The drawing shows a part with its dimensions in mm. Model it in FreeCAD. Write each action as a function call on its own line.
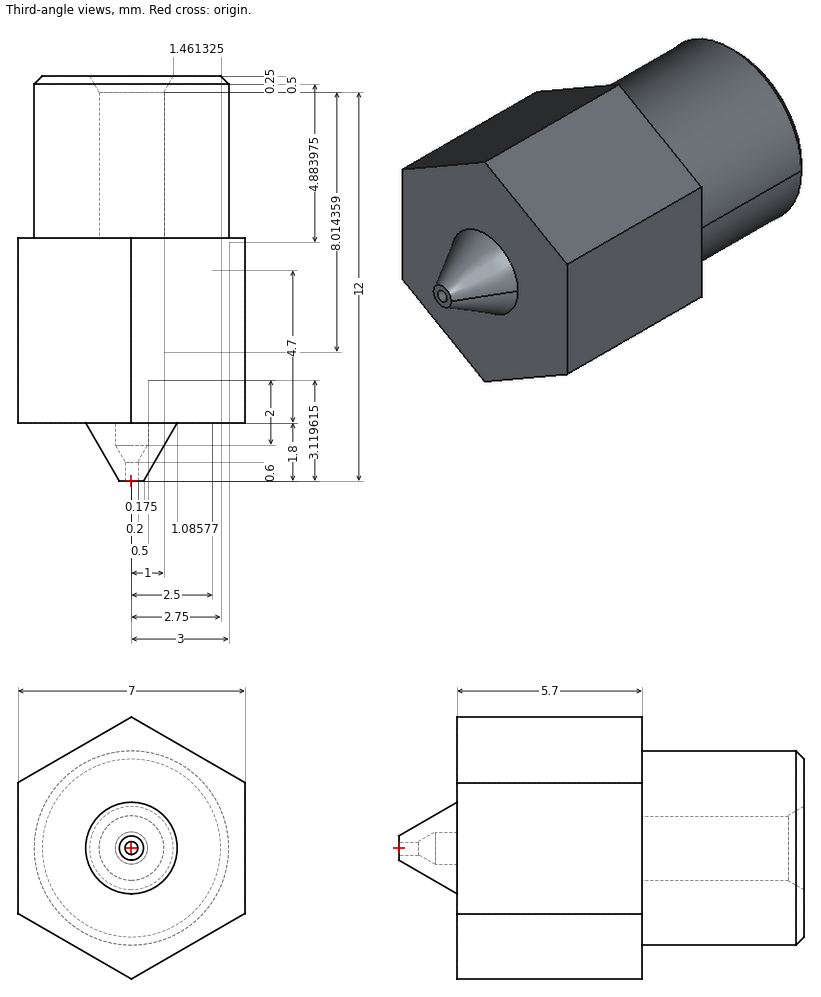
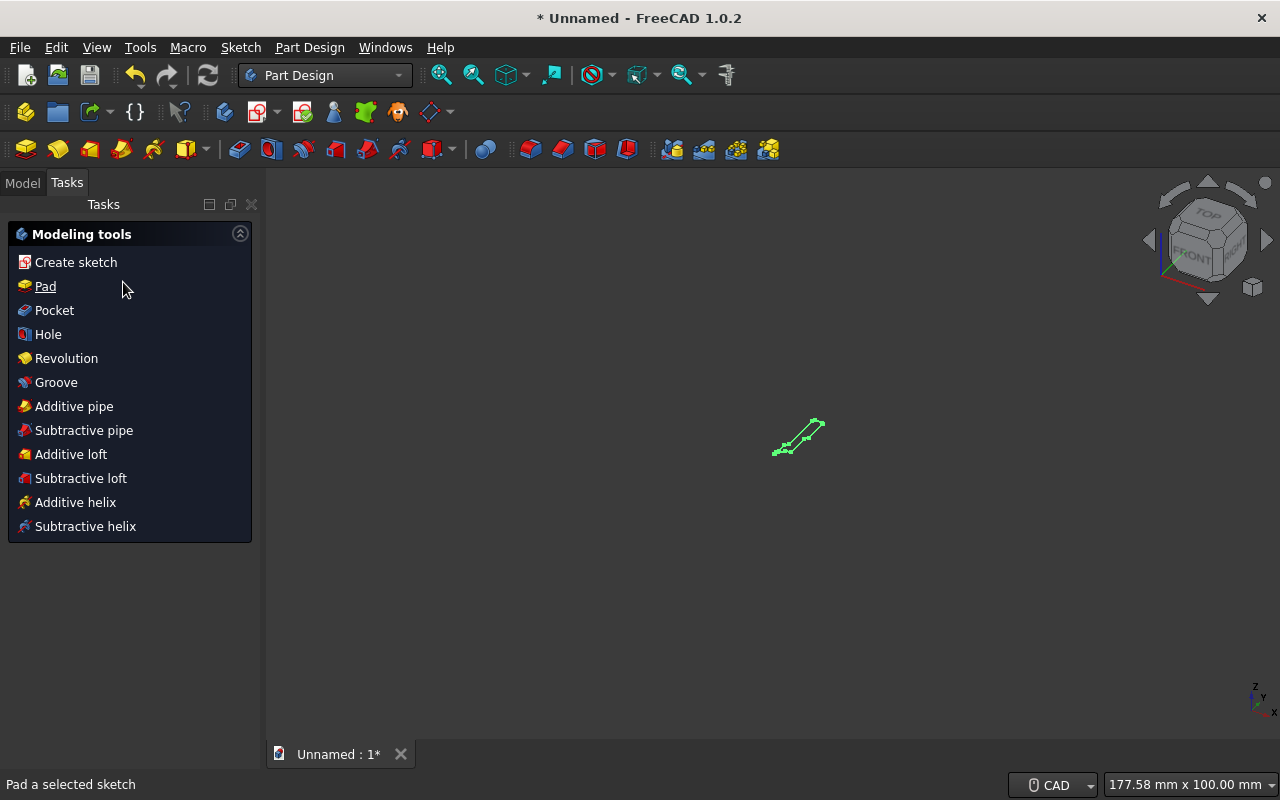
click(58, 150)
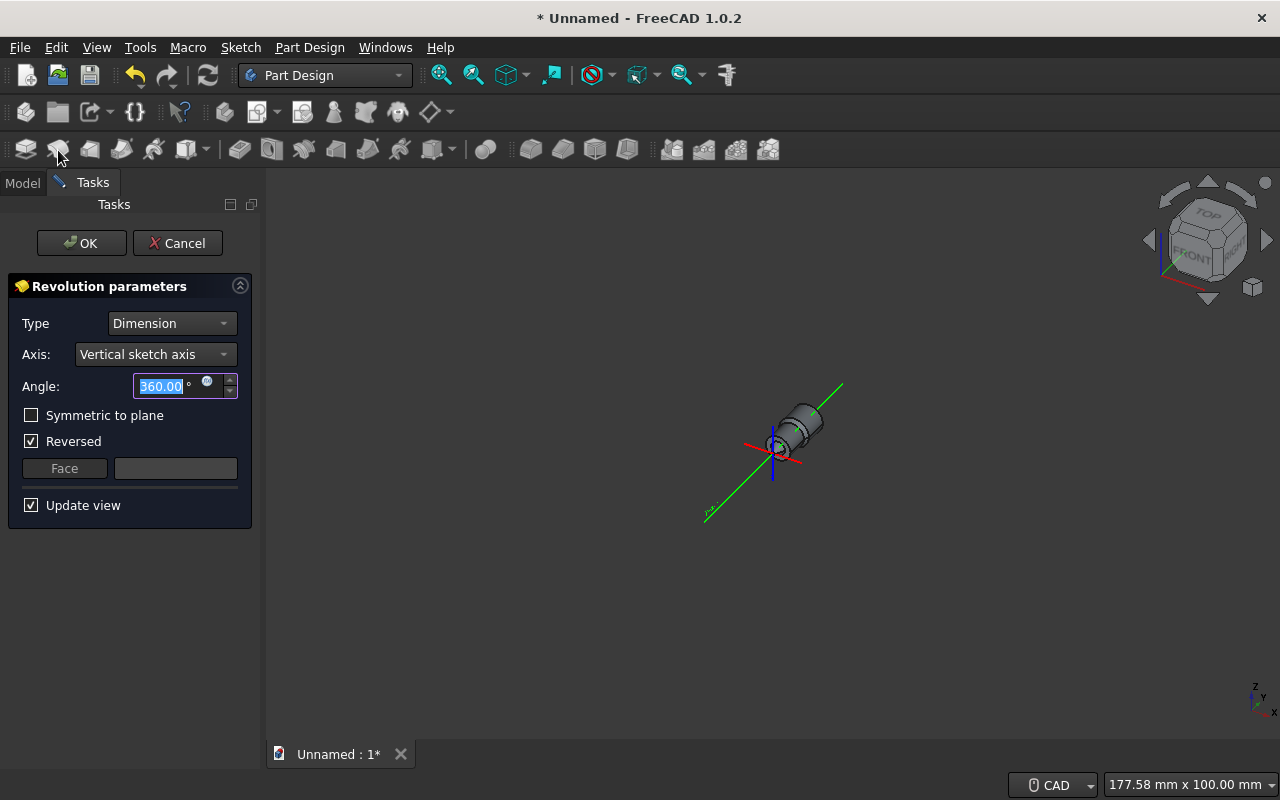
click(82, 243)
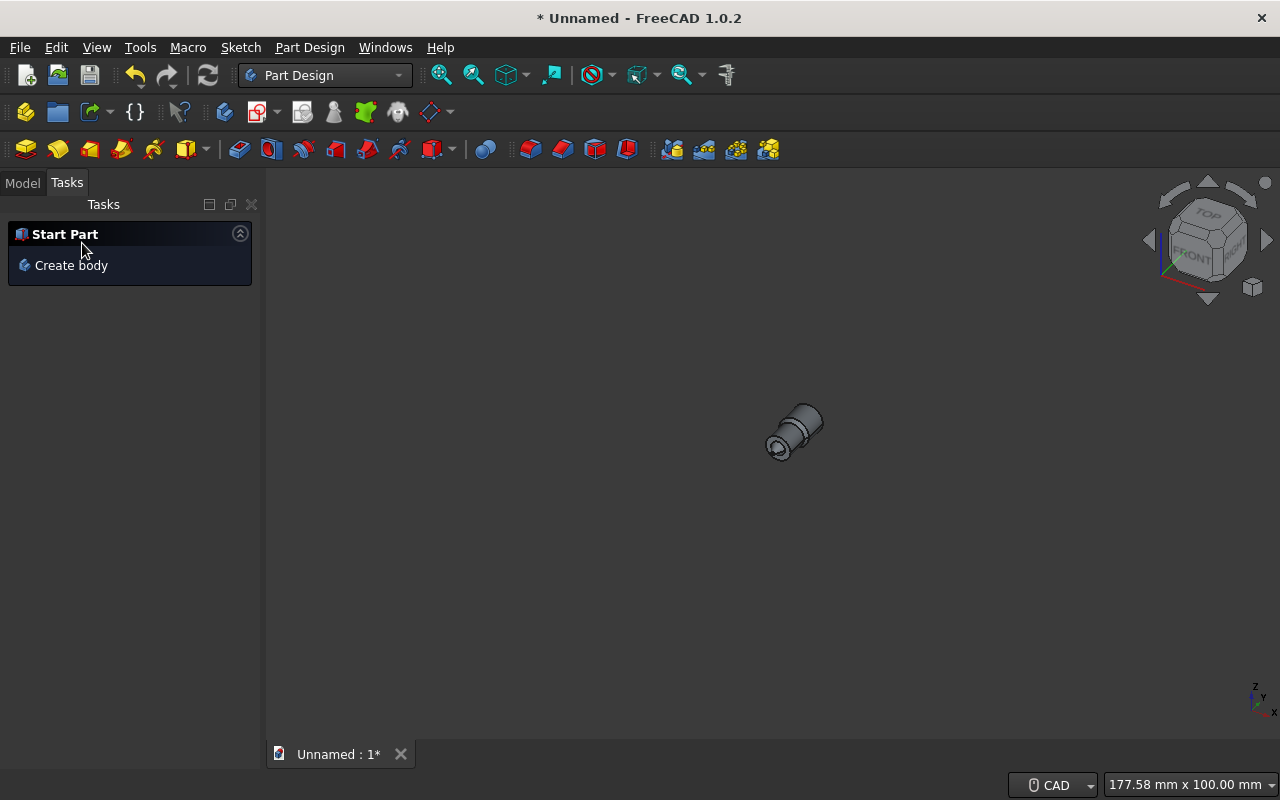
click(442, 76)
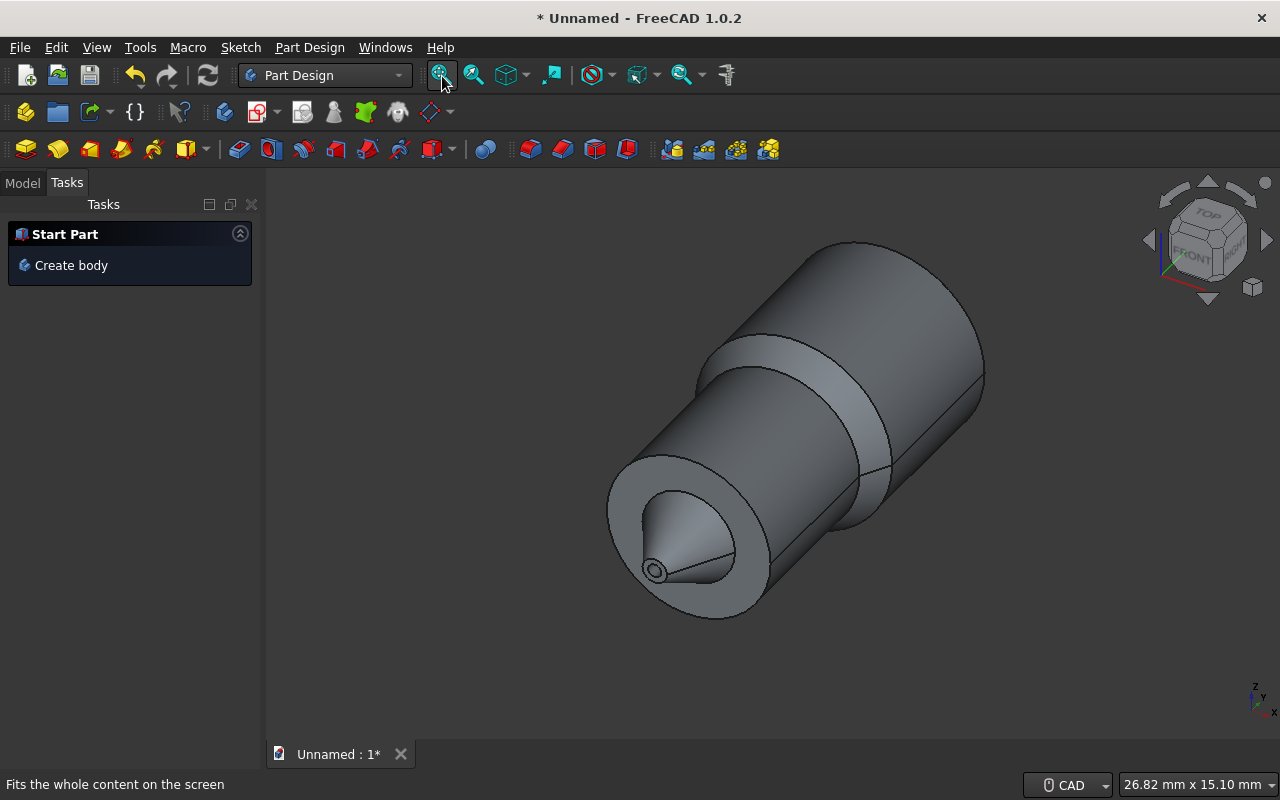
click(736, 507)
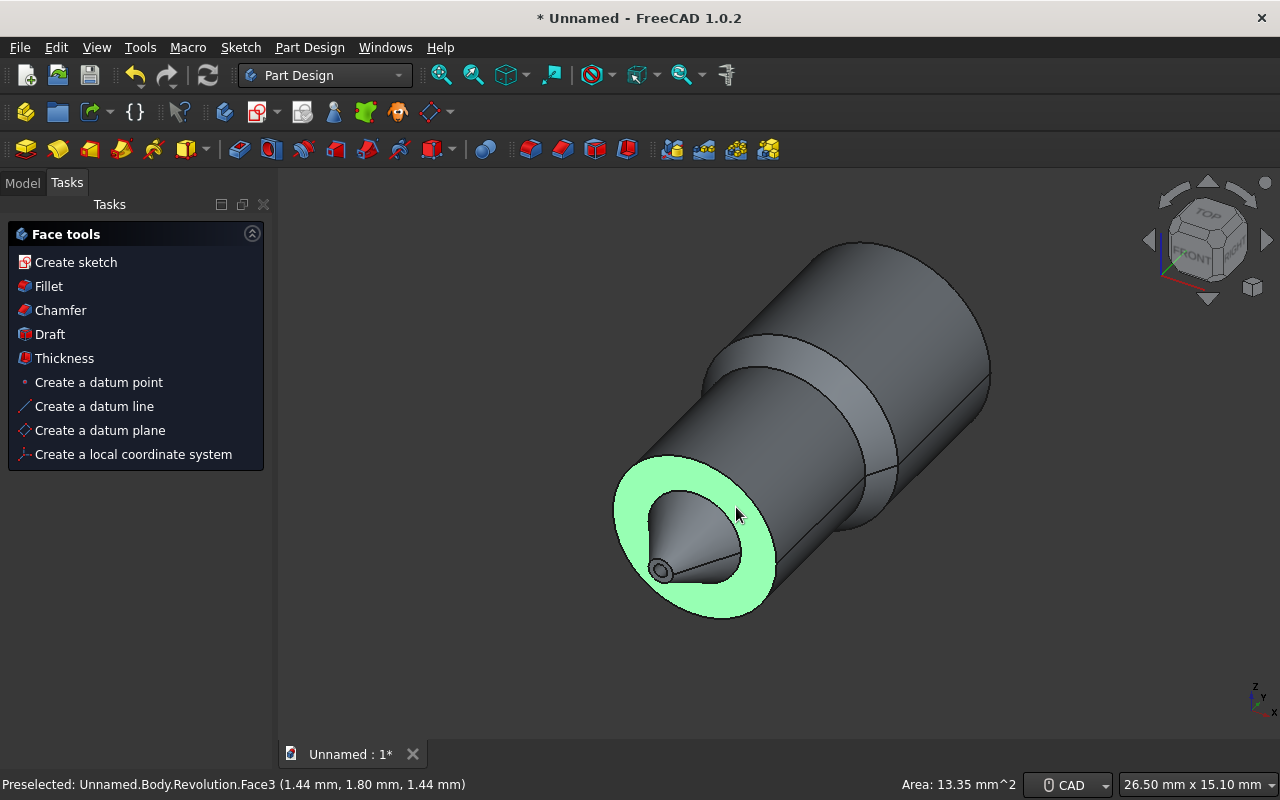
click(258, 112)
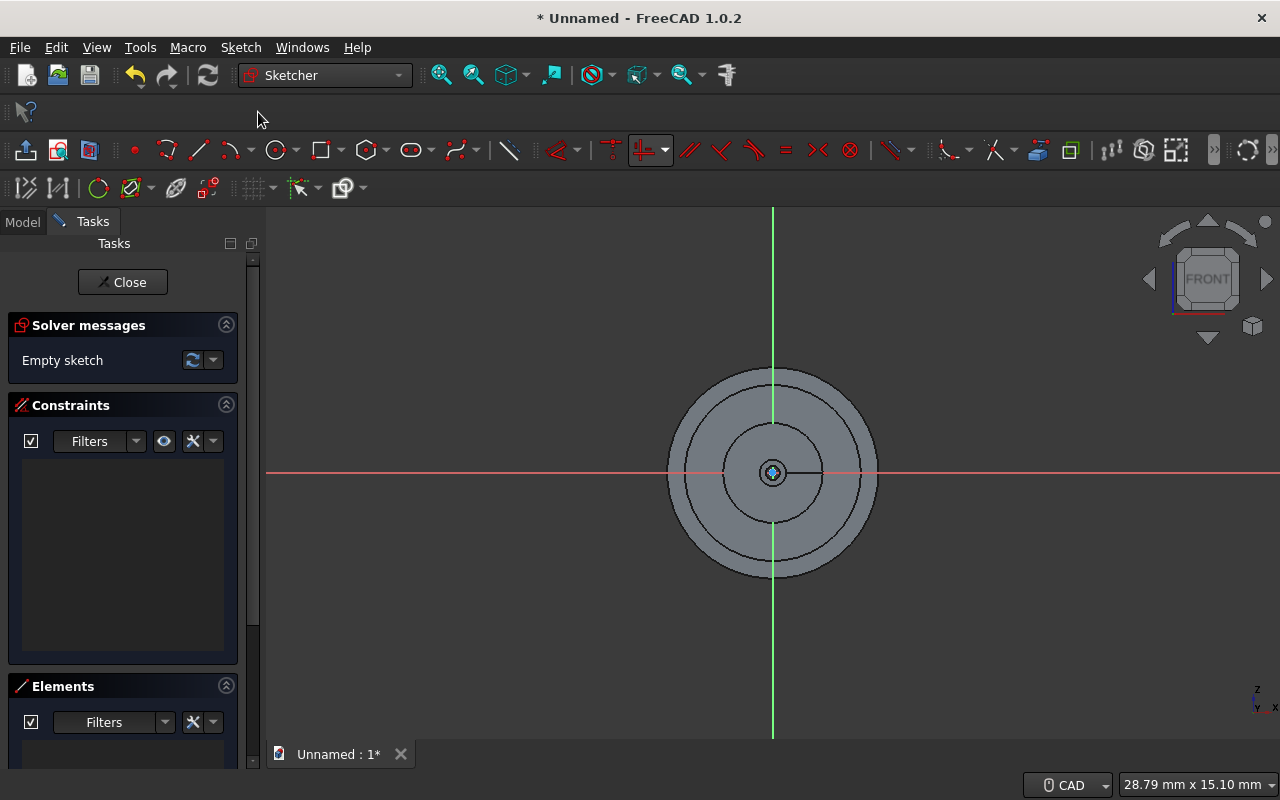
click(366, 150)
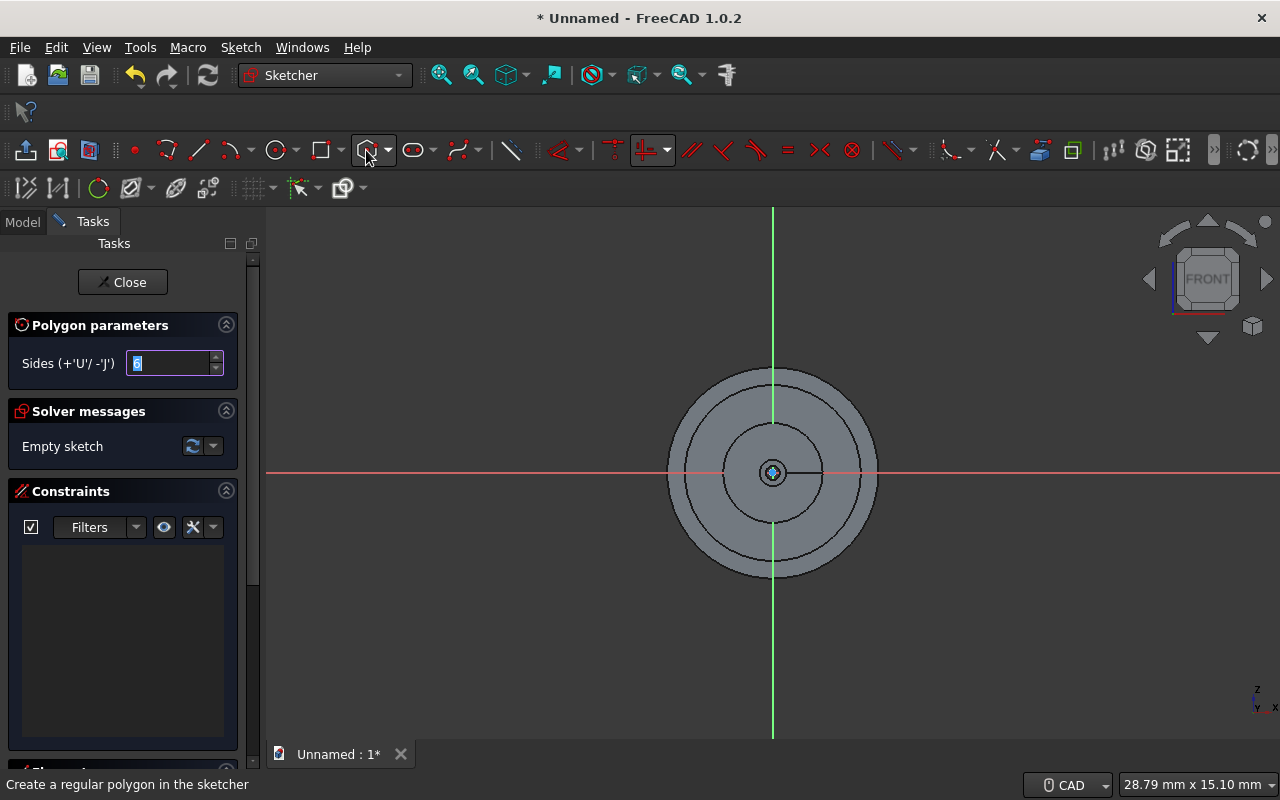
click(773, 473)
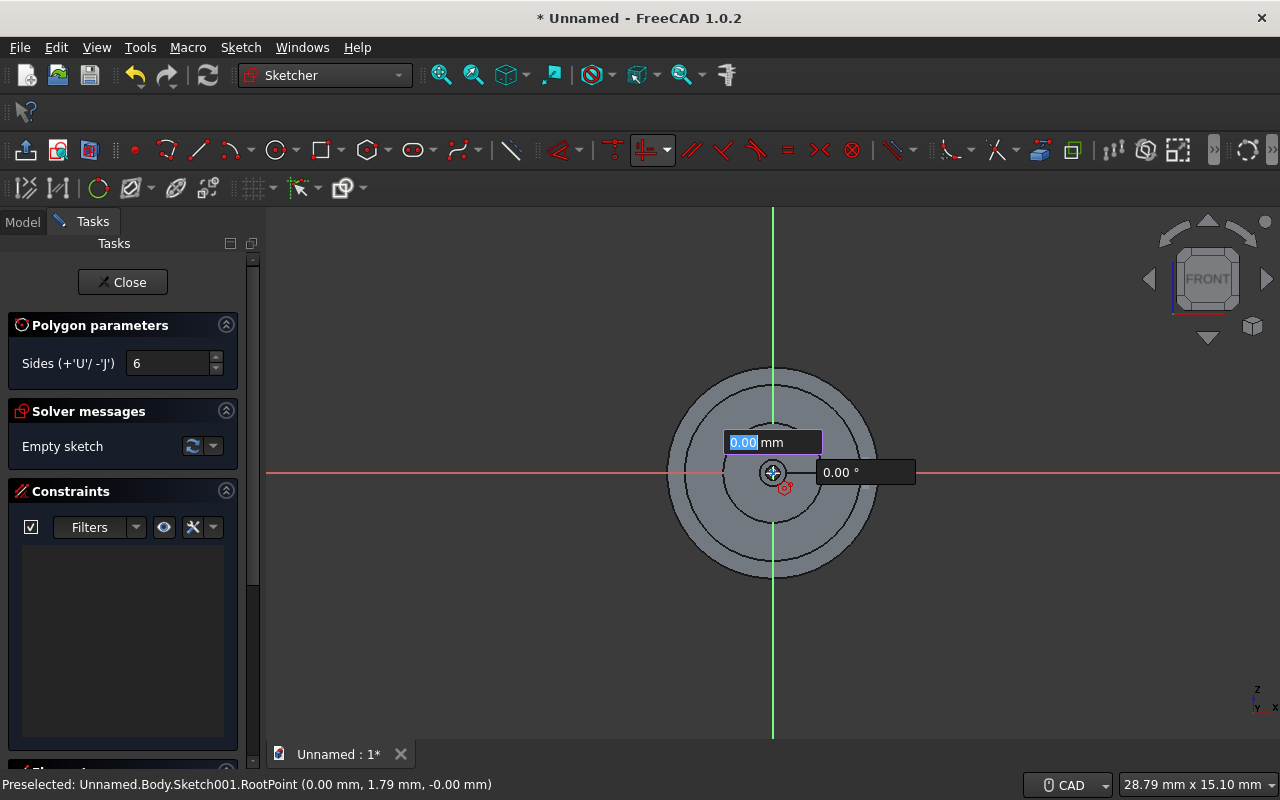
click(773, 331)
right_click(773, 331)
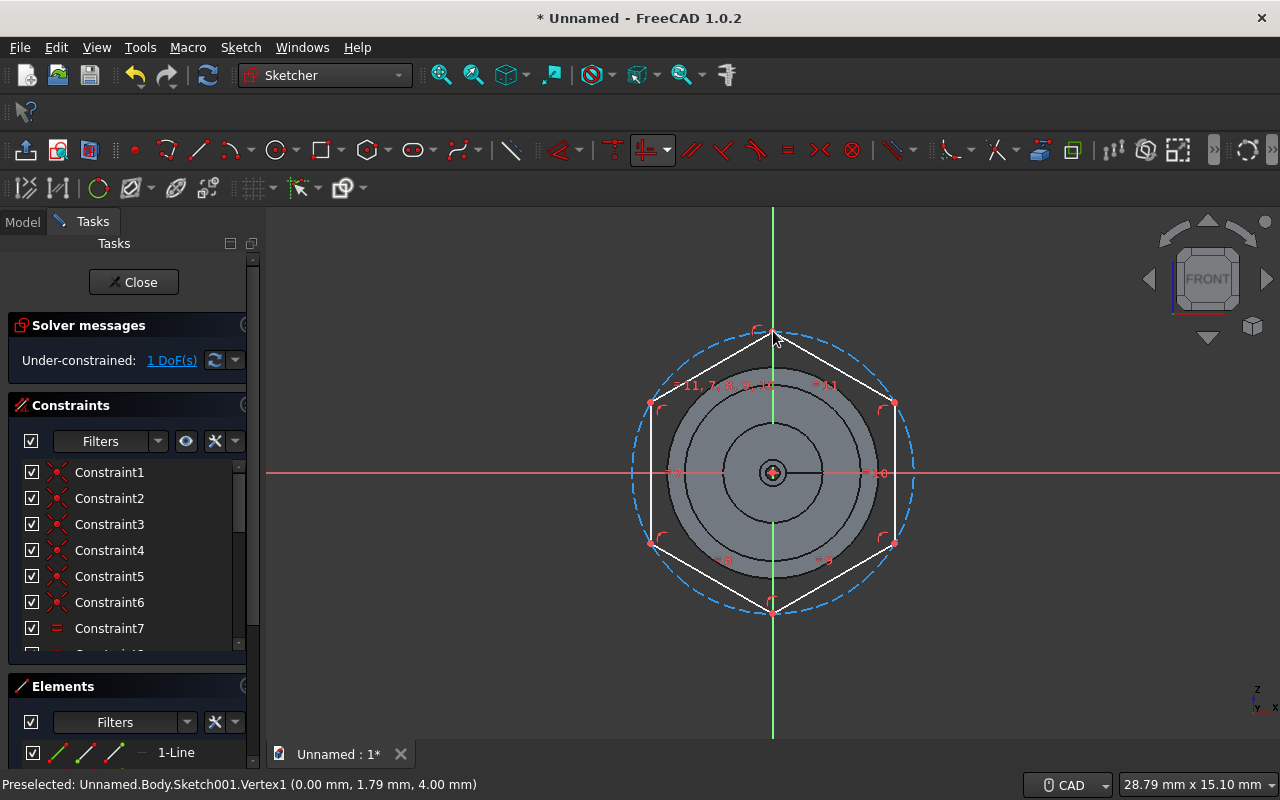
click(558, 150)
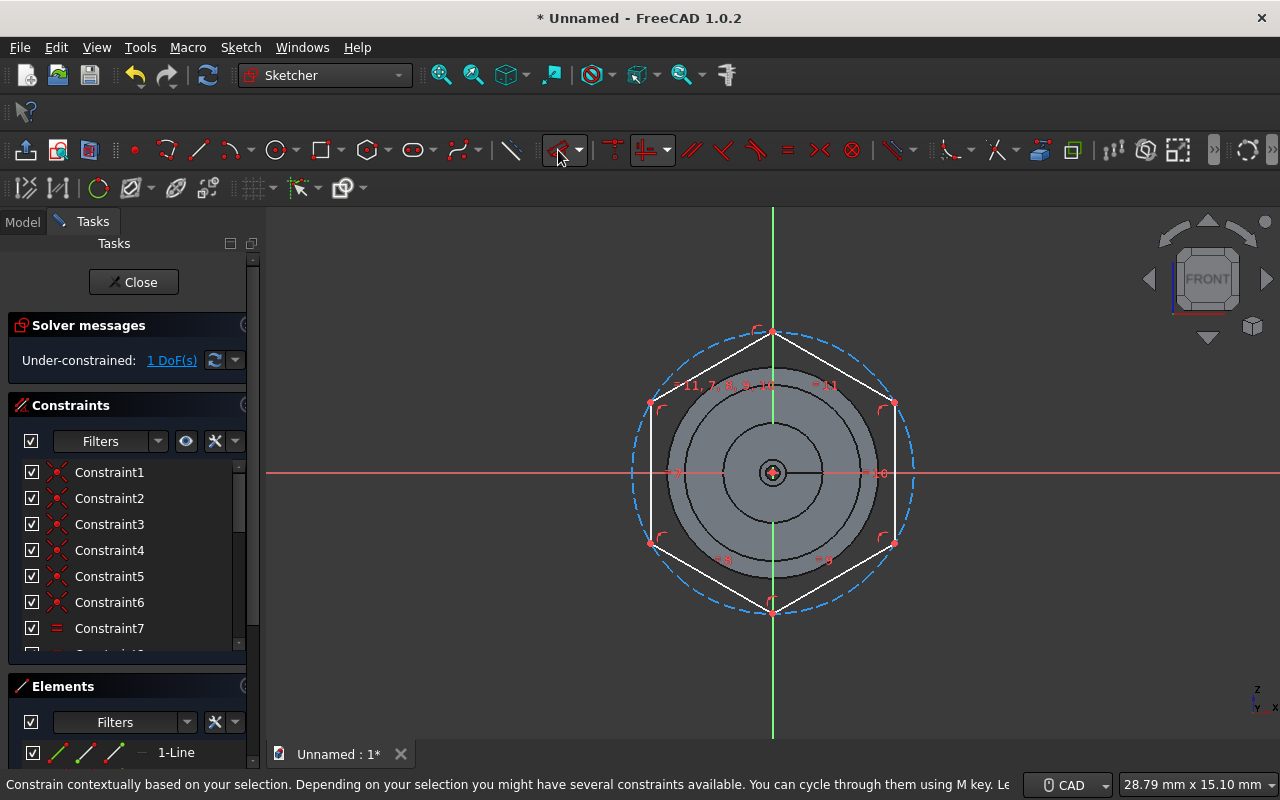
click(651, 403)